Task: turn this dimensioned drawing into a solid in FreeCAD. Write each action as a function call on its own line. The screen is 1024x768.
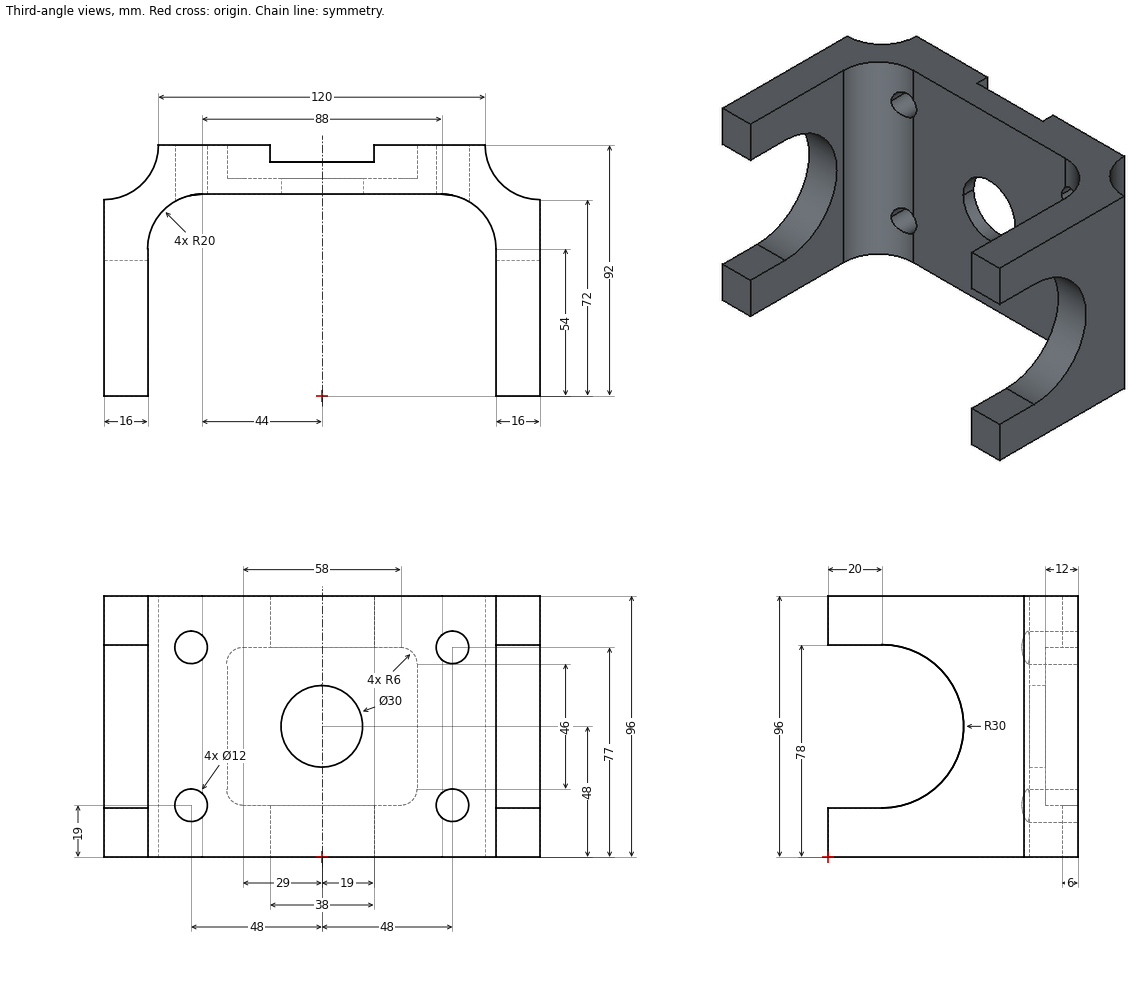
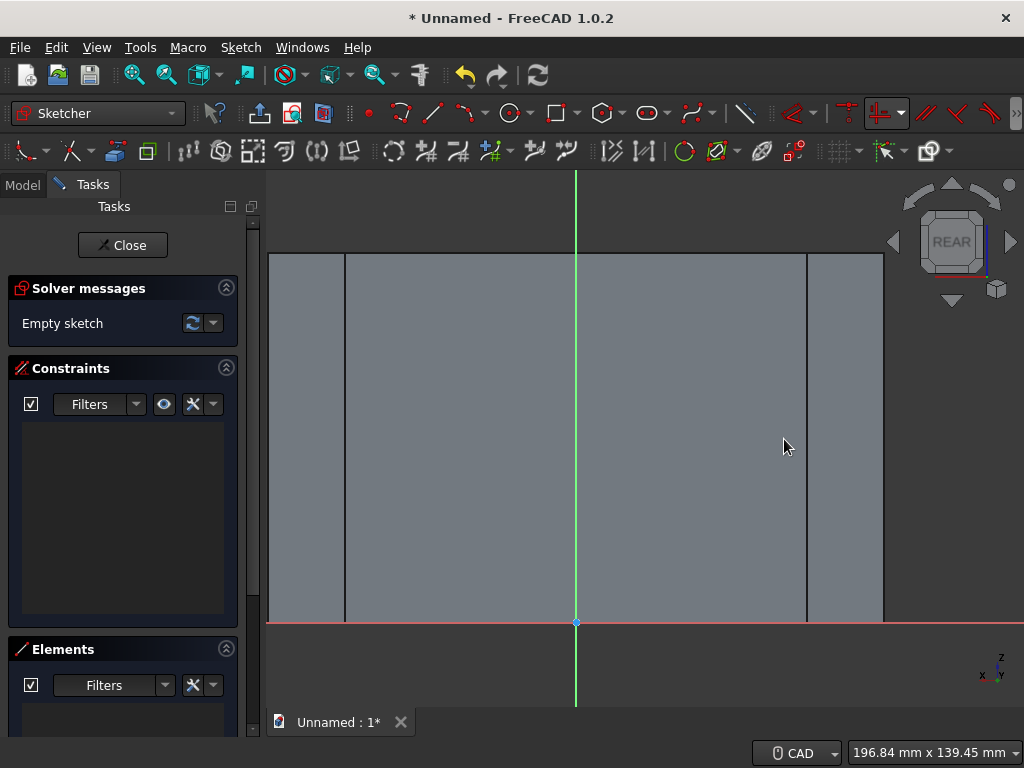
click(556, 114)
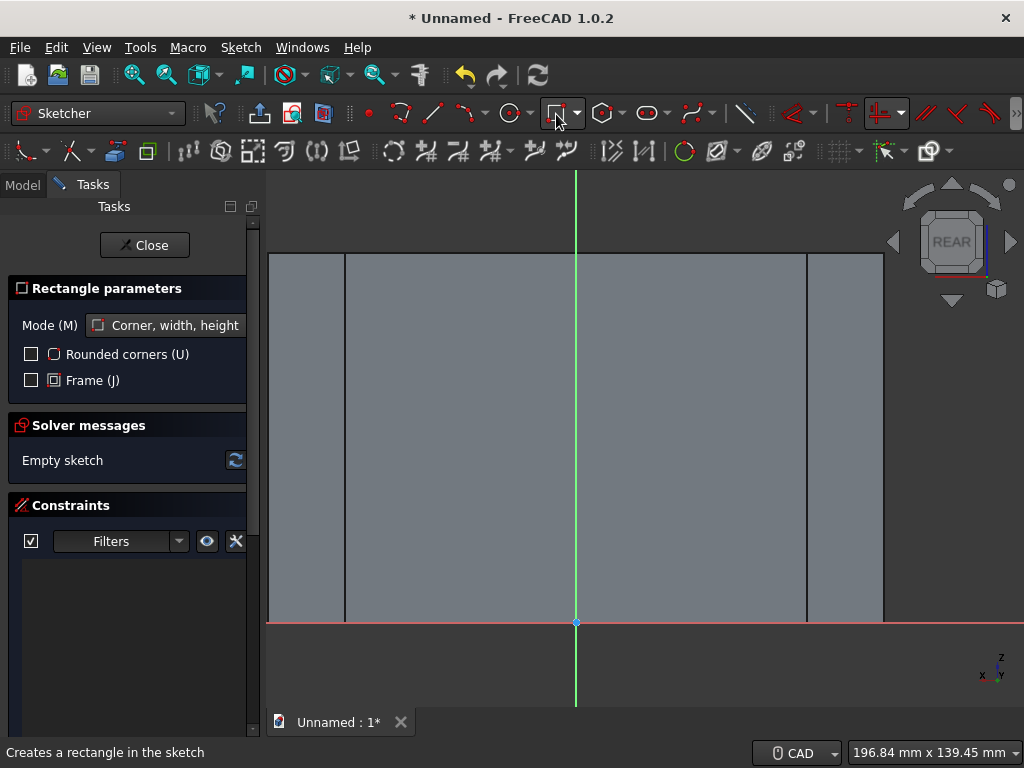
click(503, 253)
click(649, 623)
key(Escape)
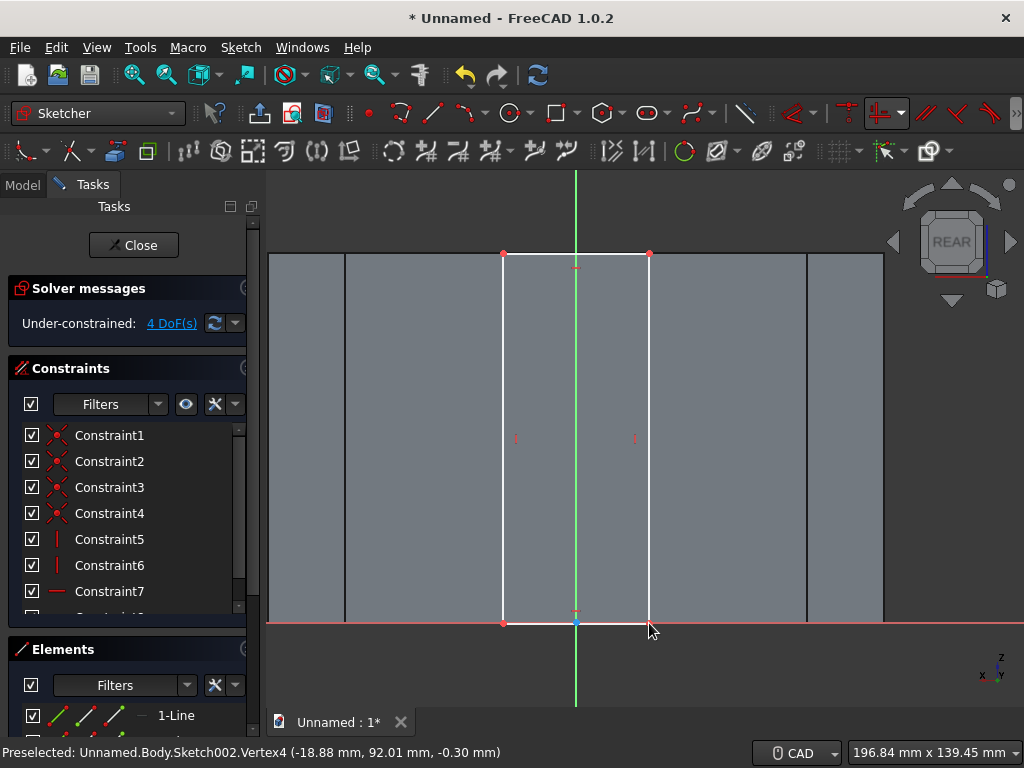
click(503, 624)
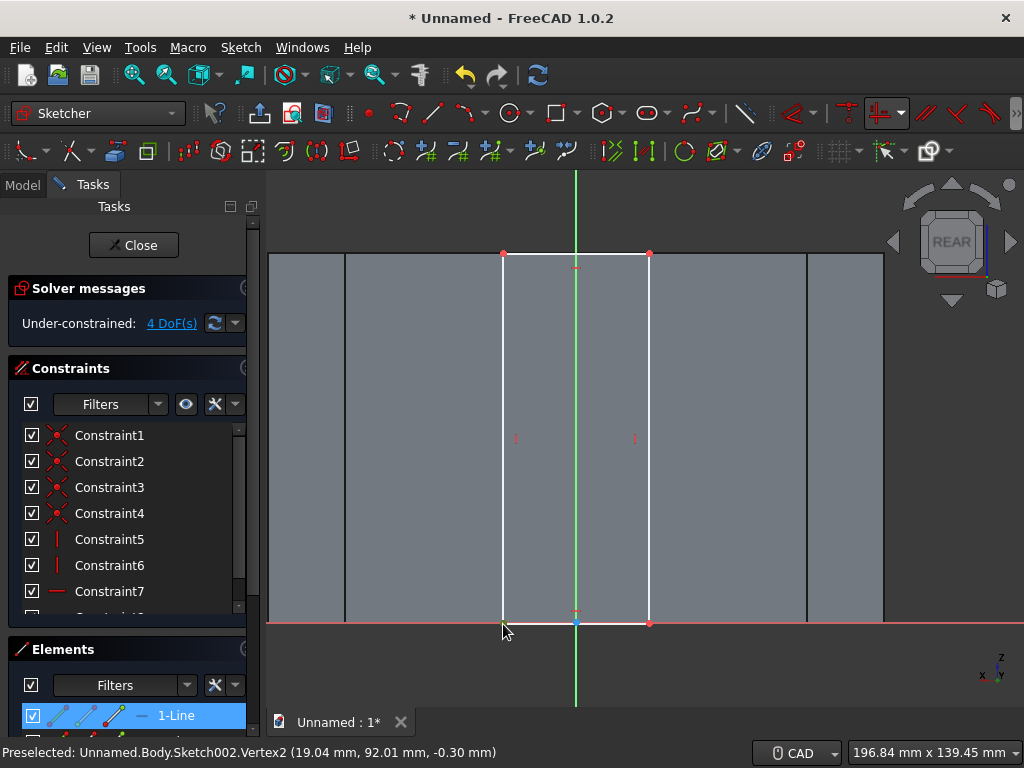
click(334, 623)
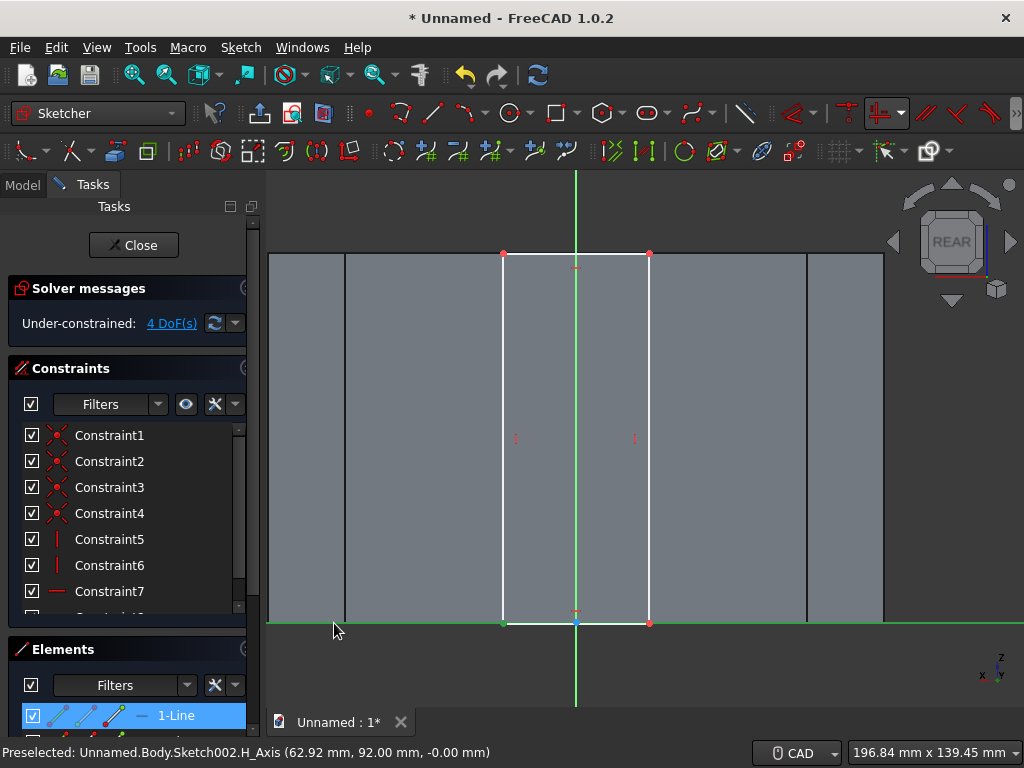
click(848, 114)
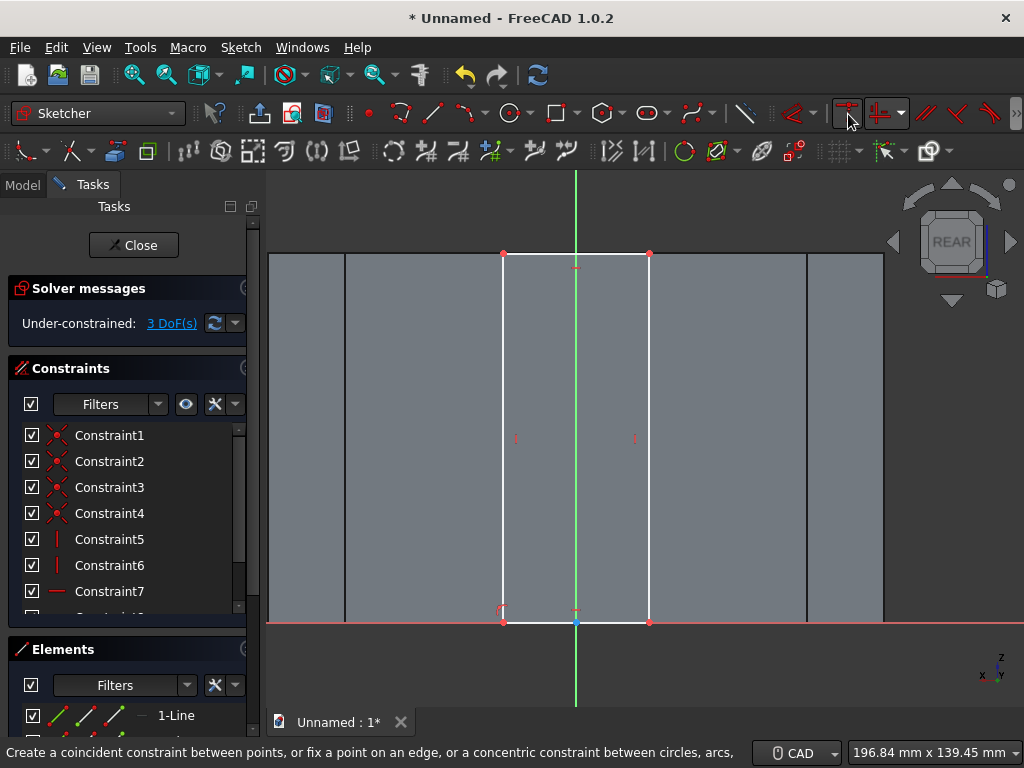
click(792, 114)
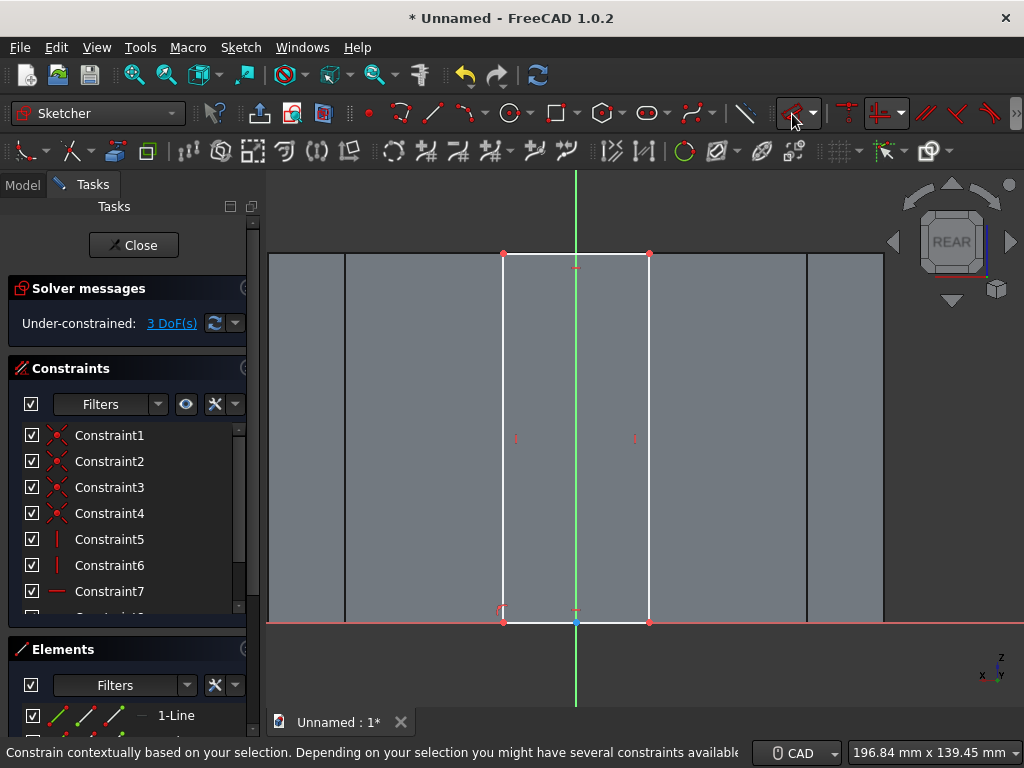
click(503, 365)
click(469, 438)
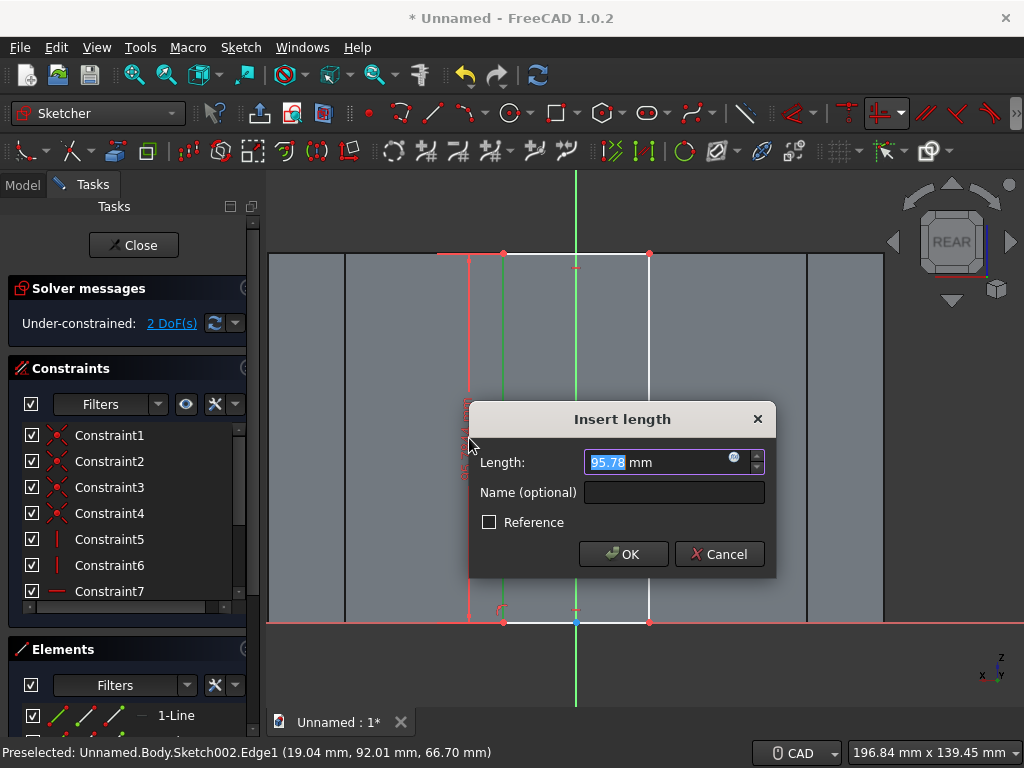
text(96)
key(Return)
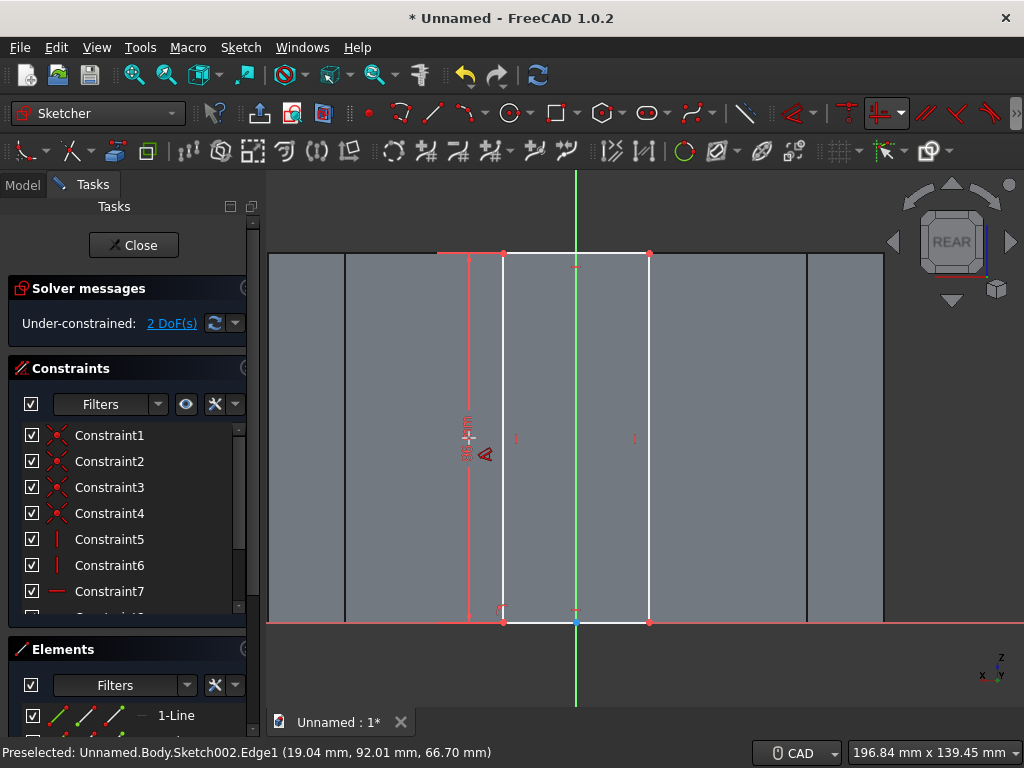
click(547, 623)
click(542, 657)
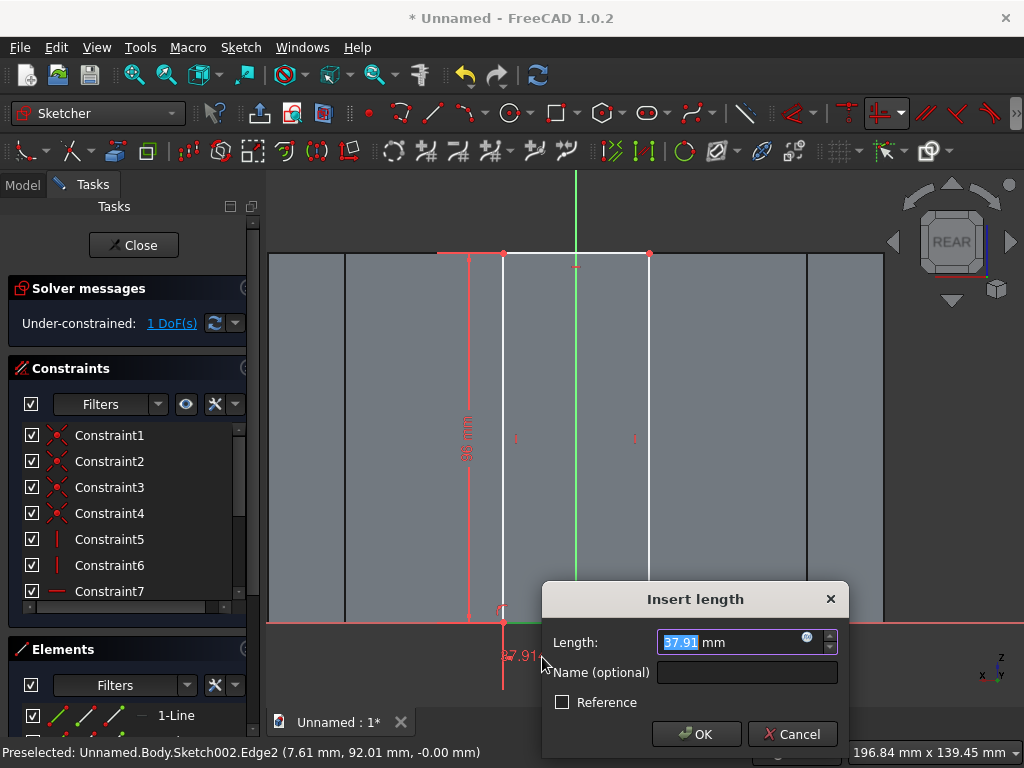
text(38)
key(Return)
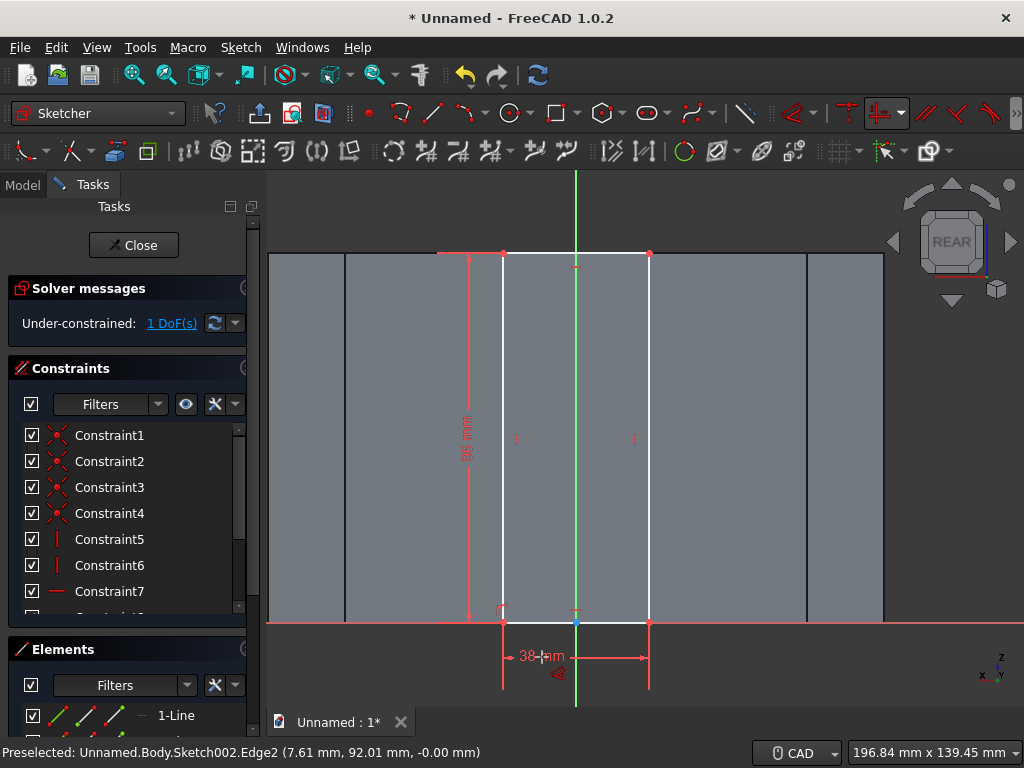
click(503, 253)
click(540, 219)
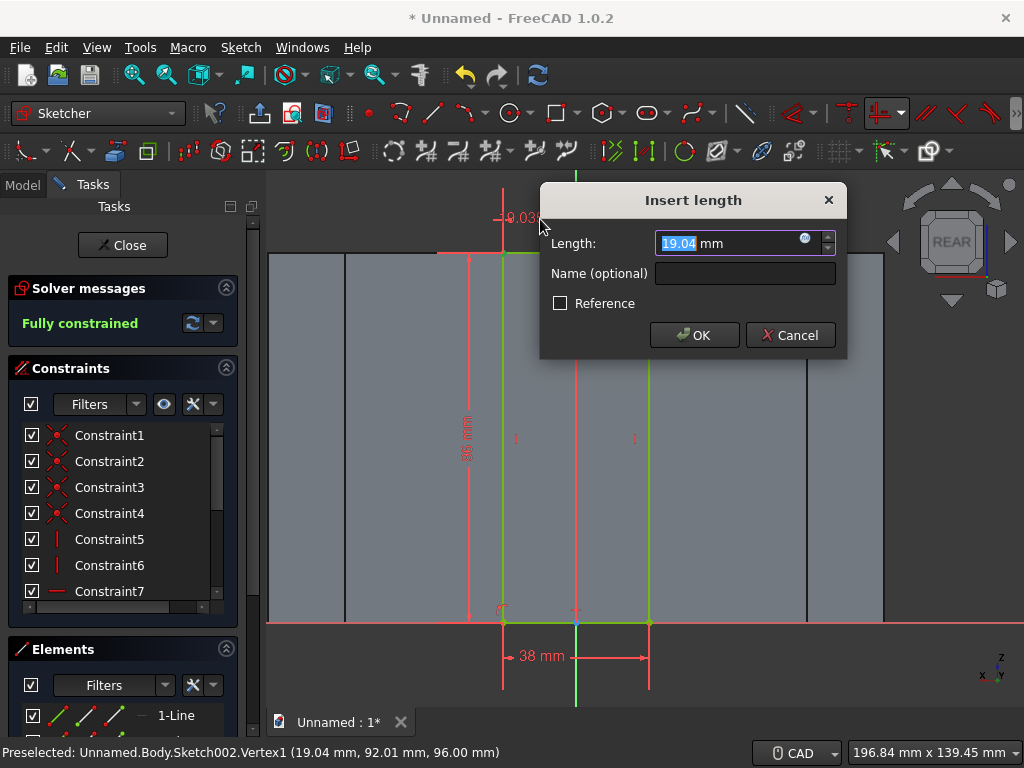
text(19)
key(Return)
key(Escape)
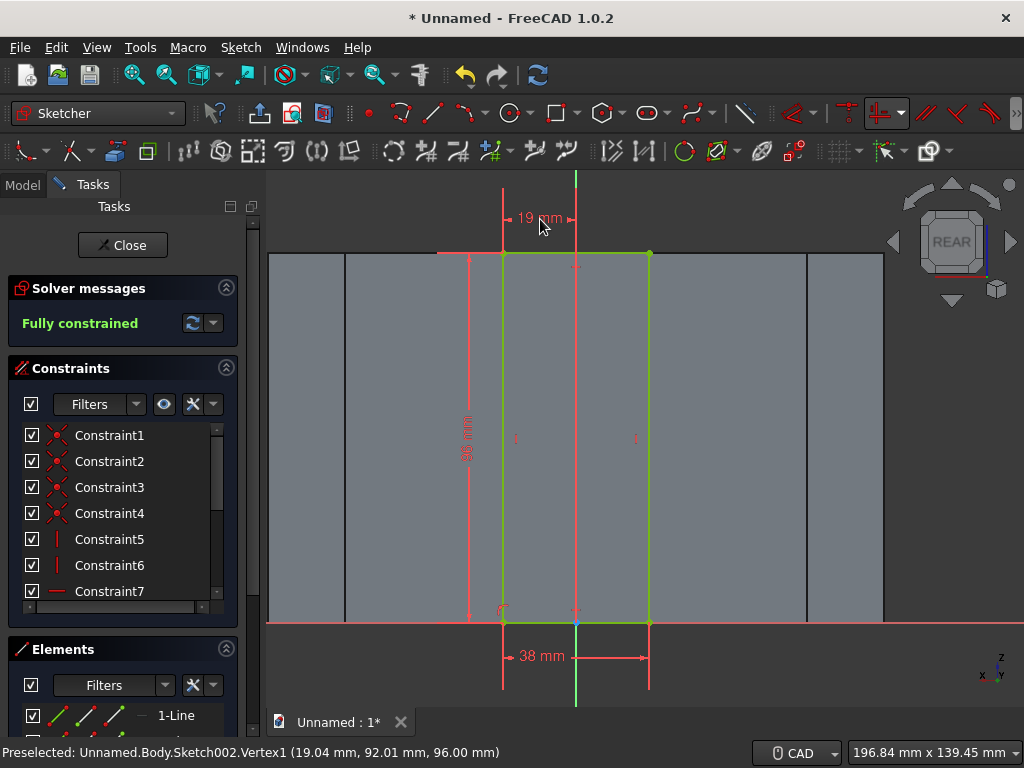
click(123, 245)